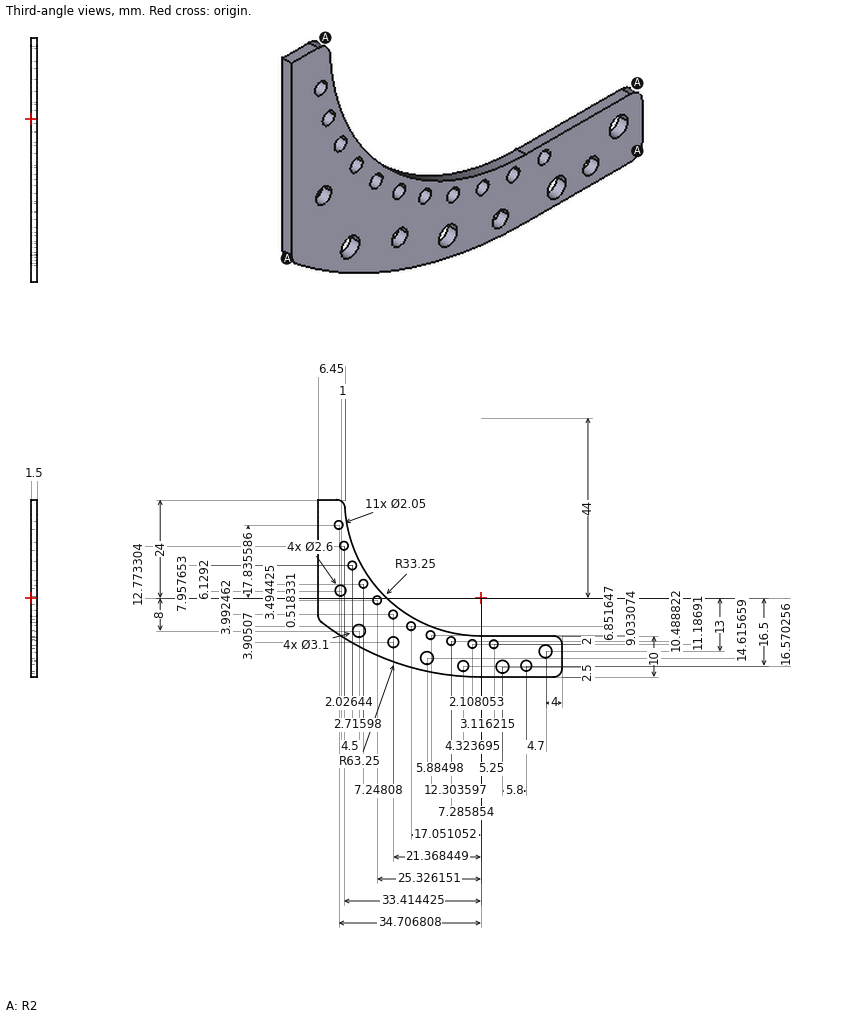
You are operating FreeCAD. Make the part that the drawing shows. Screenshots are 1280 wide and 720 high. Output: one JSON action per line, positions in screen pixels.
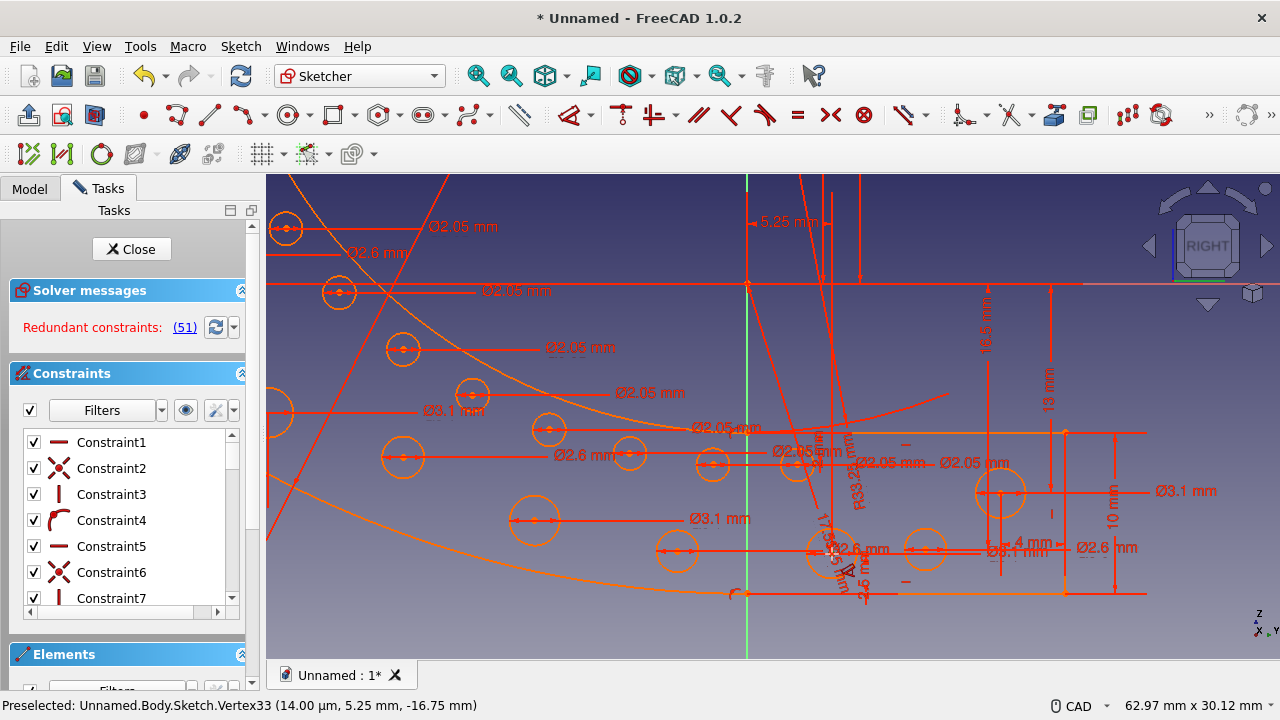
{"action": "left_click", "coordinate": [926, 550]}
{"action": "left_click", "coordinate": [879, 516]}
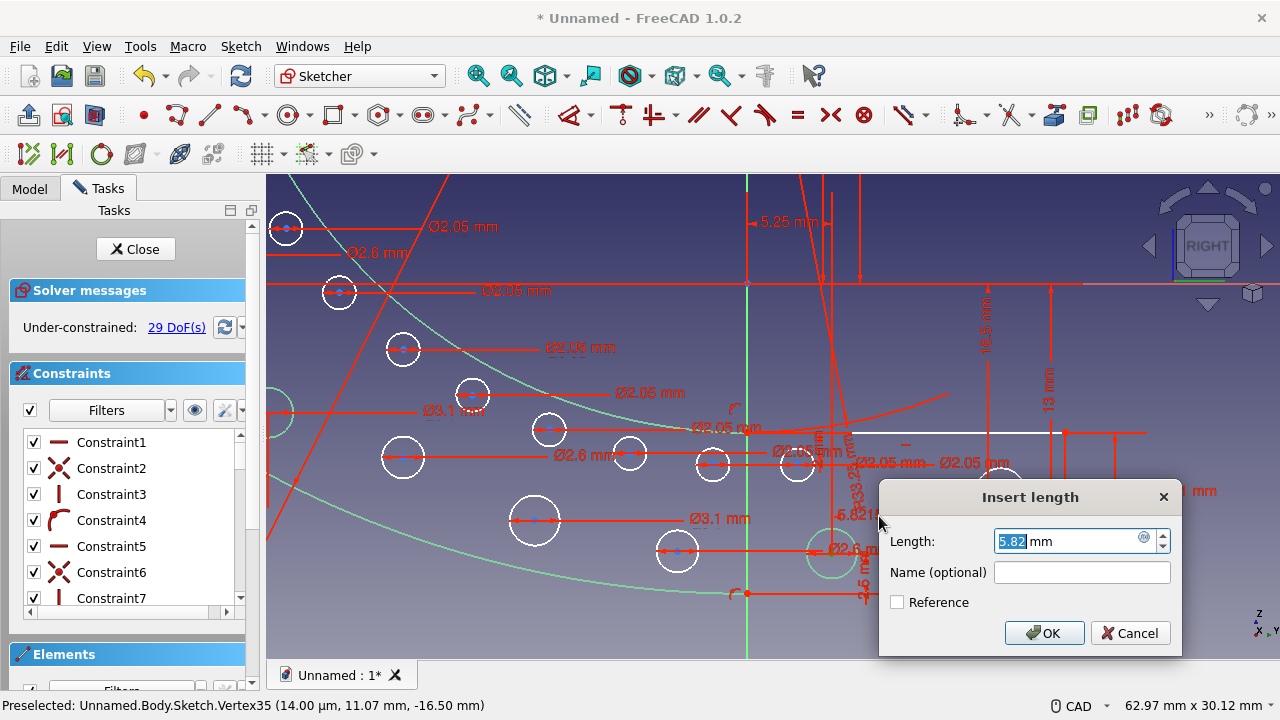
{"action": "type", "text": "5.8"}
{"action": "key", "text": "Return"}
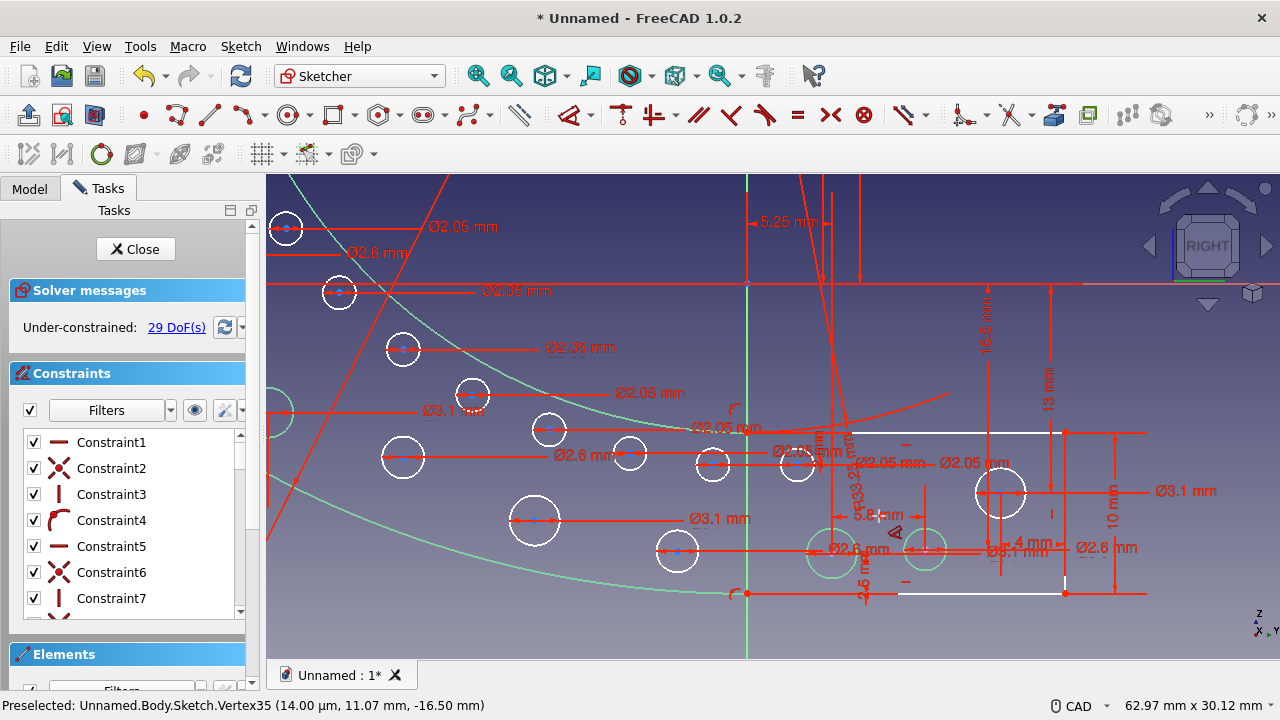
{"action": "left_click", "coordinate": [1001, 493]}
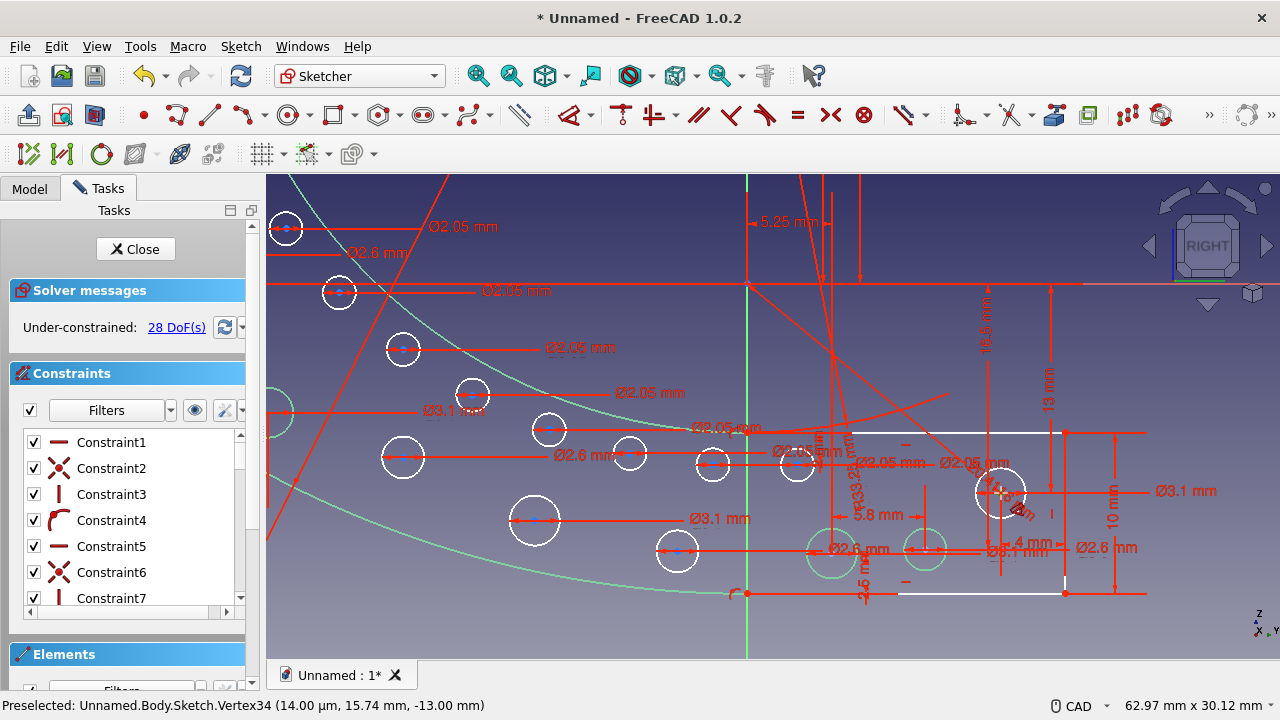
{"action": "left_click", "coordinate": [925, 550]}
{"action": "left_click", "coordinate": [963, 459]}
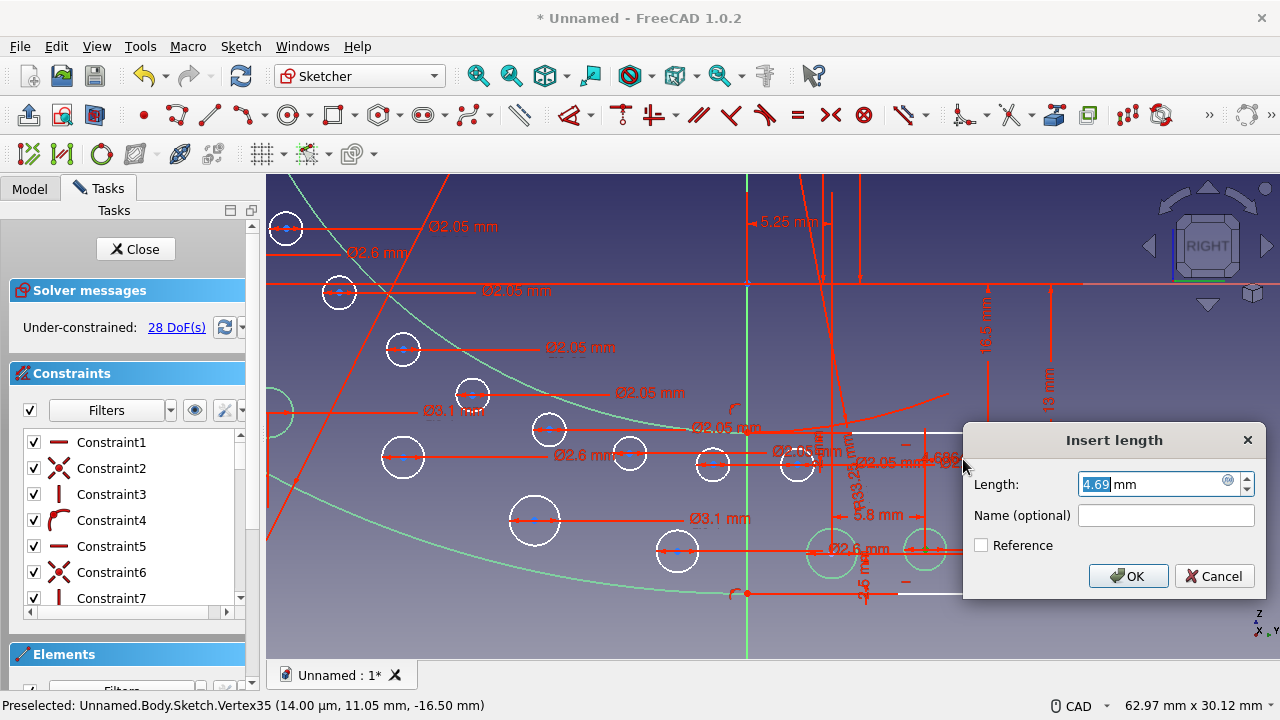
{"action": "type", "text": "4.7"}
{"action": "key", "text": "Return"}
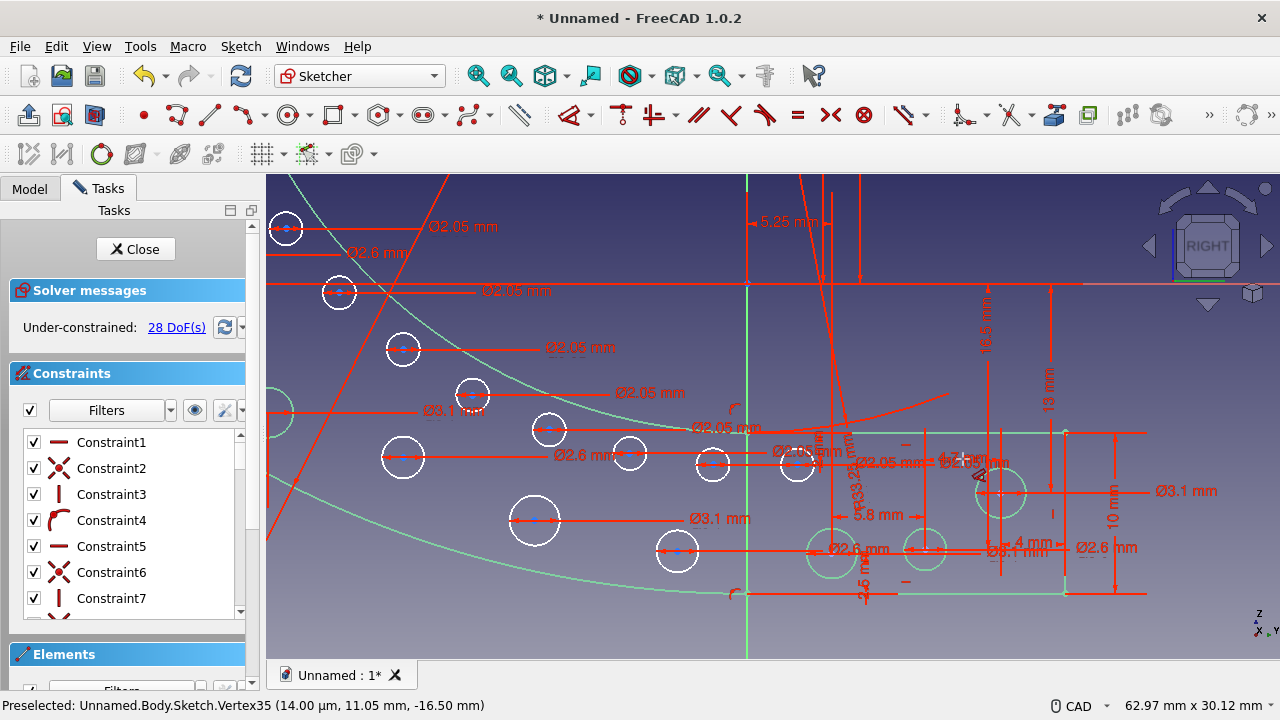
{"action": "scroll", "coordinate": [801, 556], "scroll_direction": "down", "scroll_amount": 4}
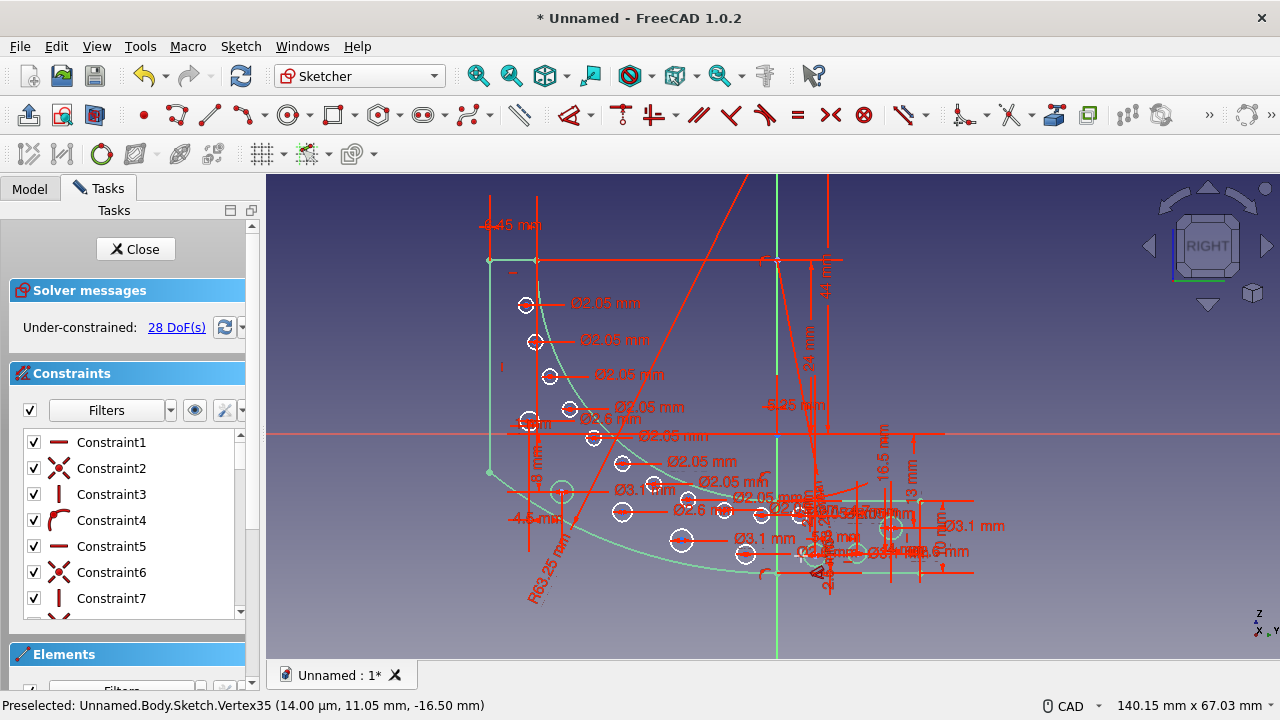
{"action": "left_click", "coordinate": [550, 377]}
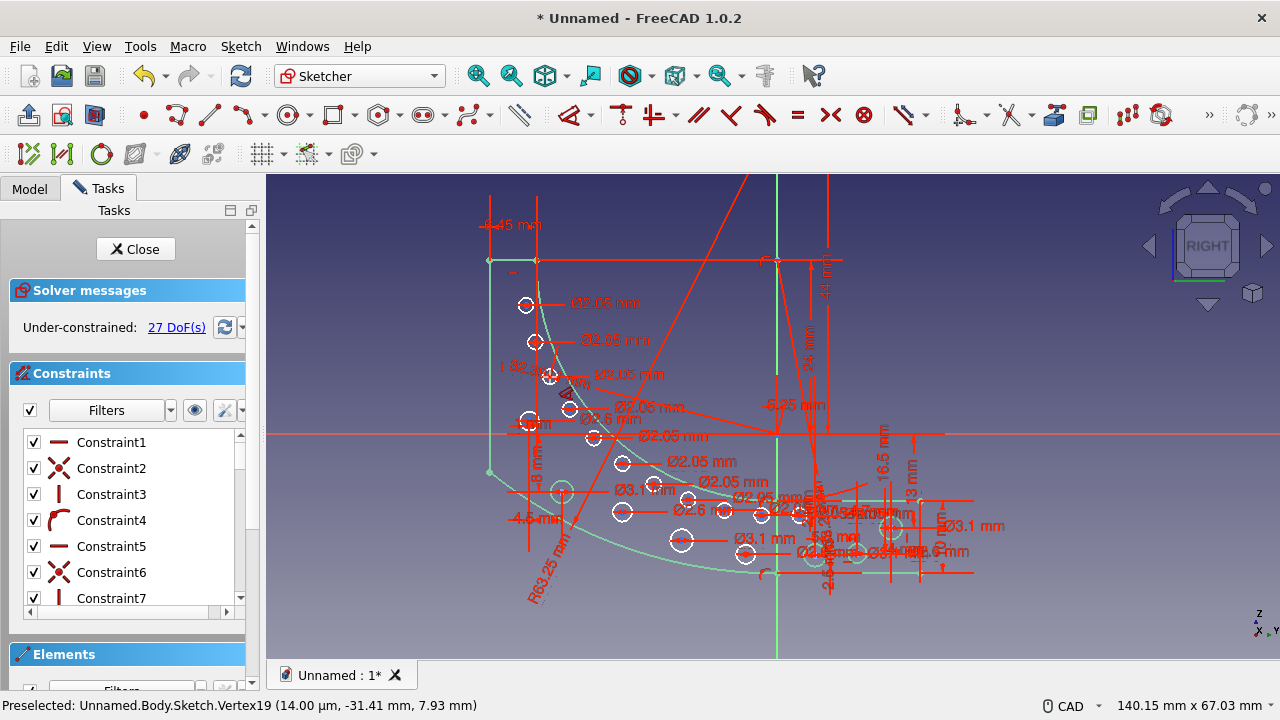
{"action": "left_click", "coordinate": [529, 421]}
{"action": "left_click", "coordinate": [471, 399]}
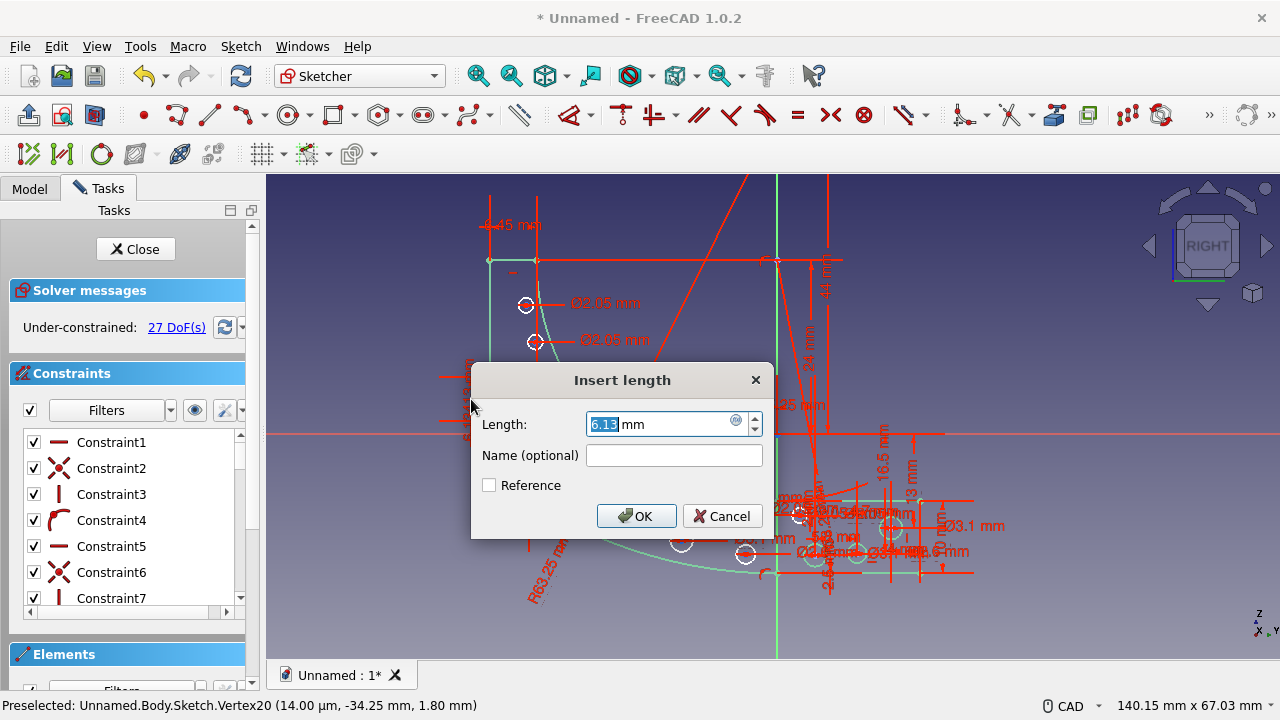
{"action": "type", "text": "6.1292"}
{"action": "key", "text": "Return"}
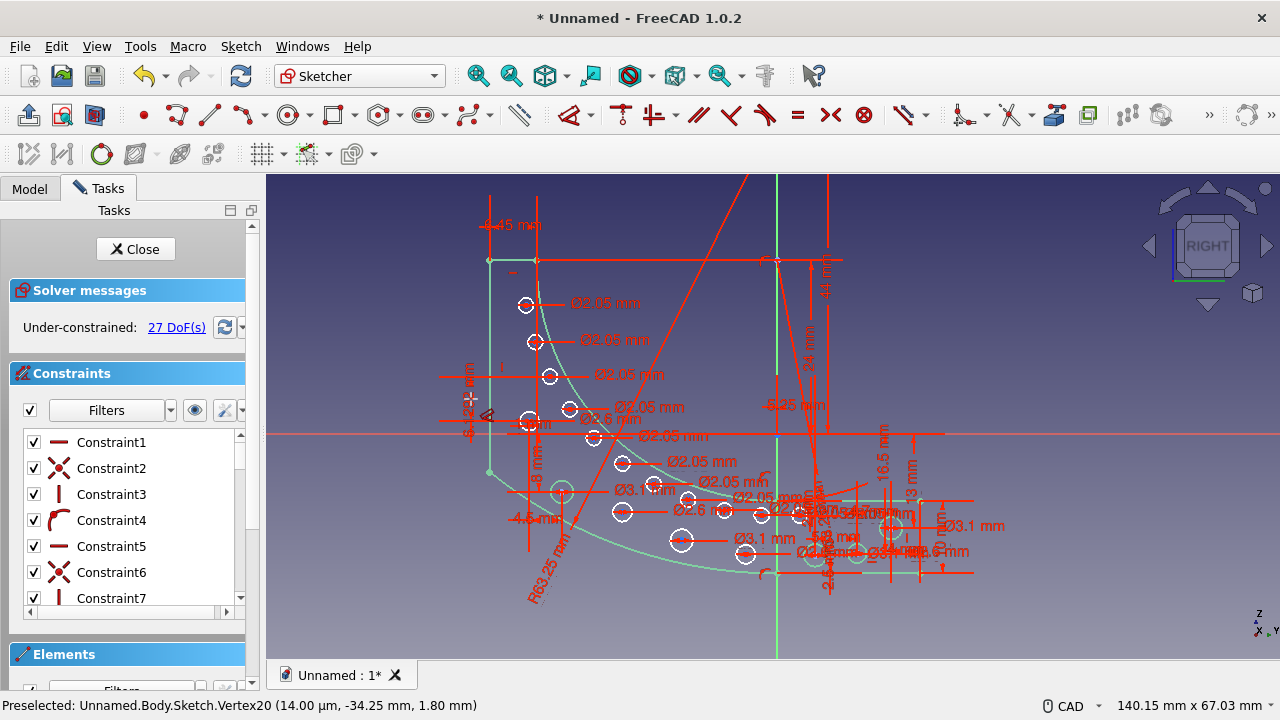
{"action": "left_click", "coordinate": [550, 377]}
{"action": "left_click", "coordinate": [811, 385]}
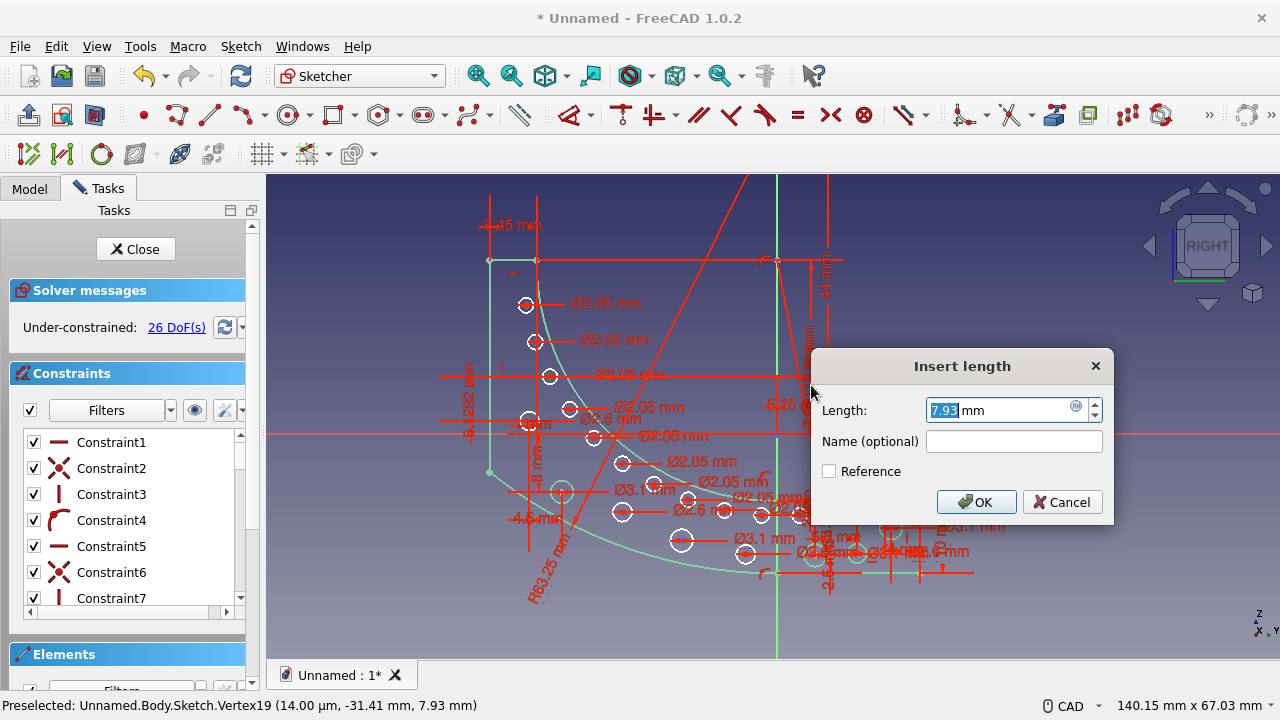
{"action": "type", "text": "7.957653"}
{"action": "key", "text": "Return"}